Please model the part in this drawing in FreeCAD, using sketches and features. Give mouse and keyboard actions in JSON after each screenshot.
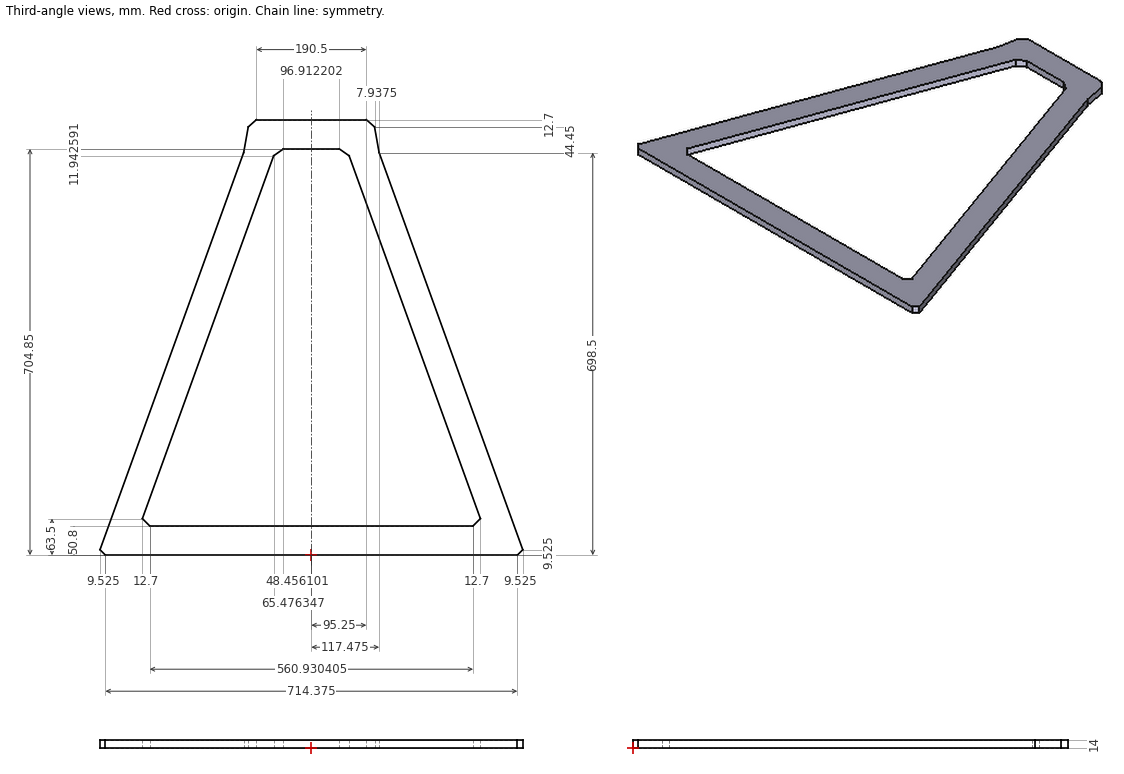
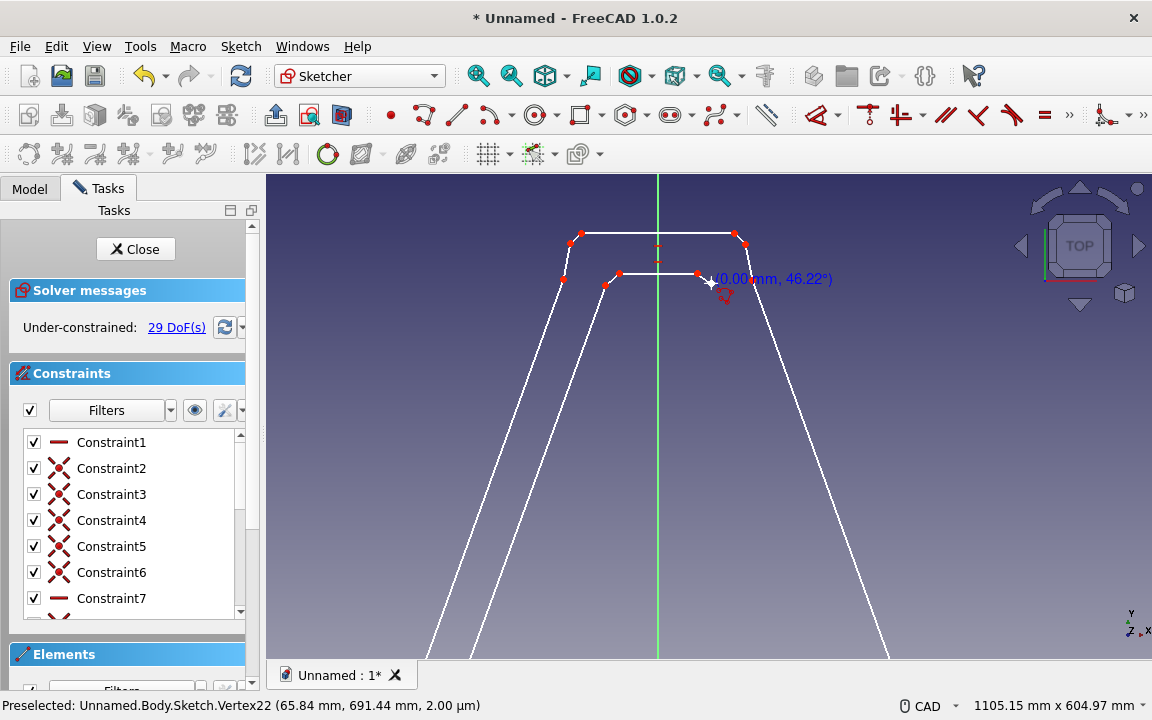
{"action": "scroll", "coordinate": [619, 272], "scroll_direction": "down", "scroll_amount": 3}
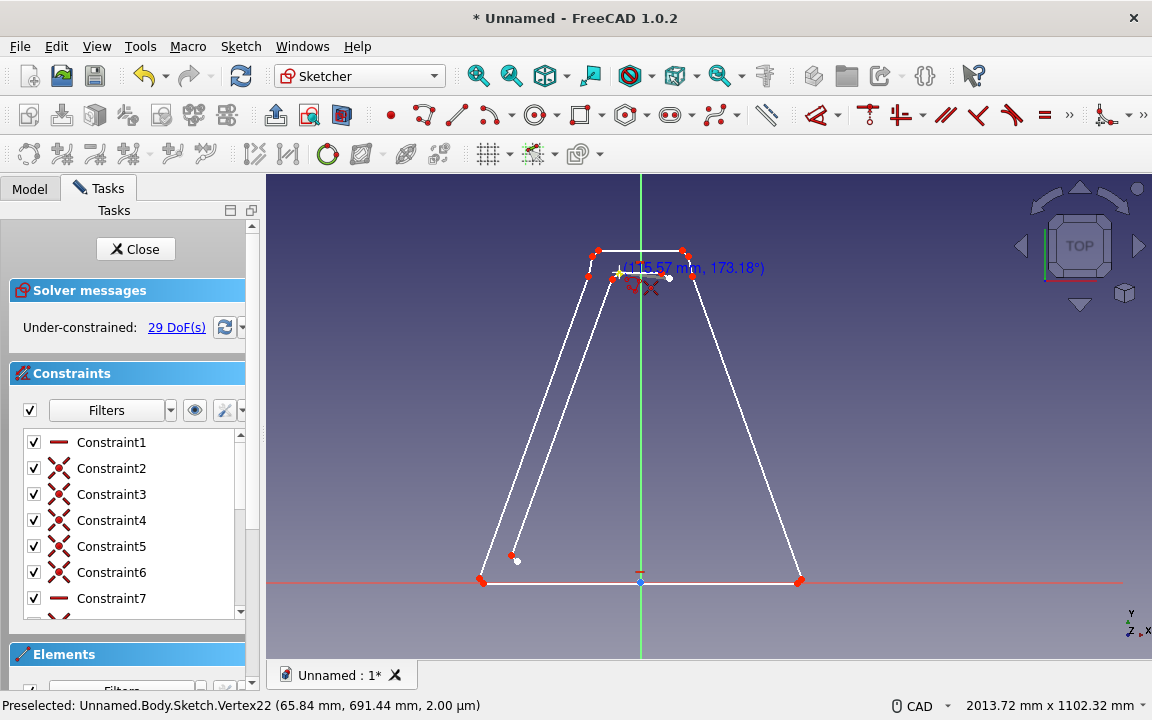
{"action": "left_click", "coordinate": [770, 555]}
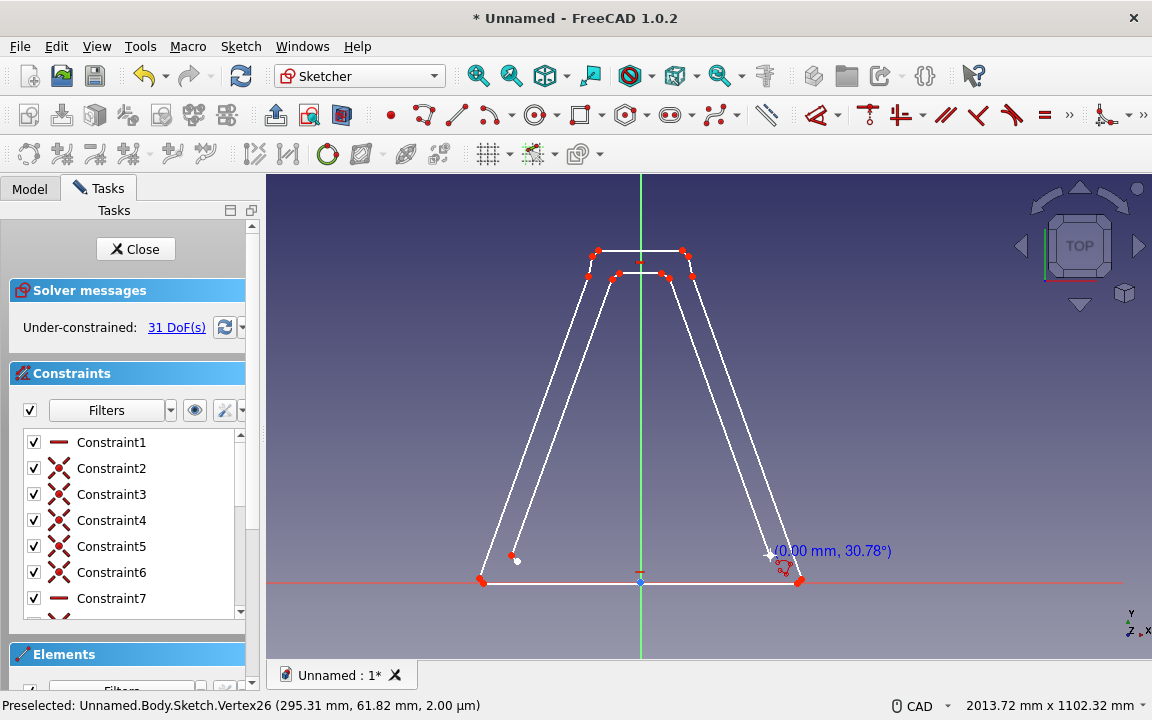
{"action": "scroll", "coordinate": [764, 561], "scroll_direction": "up", "scroll_amount": 4}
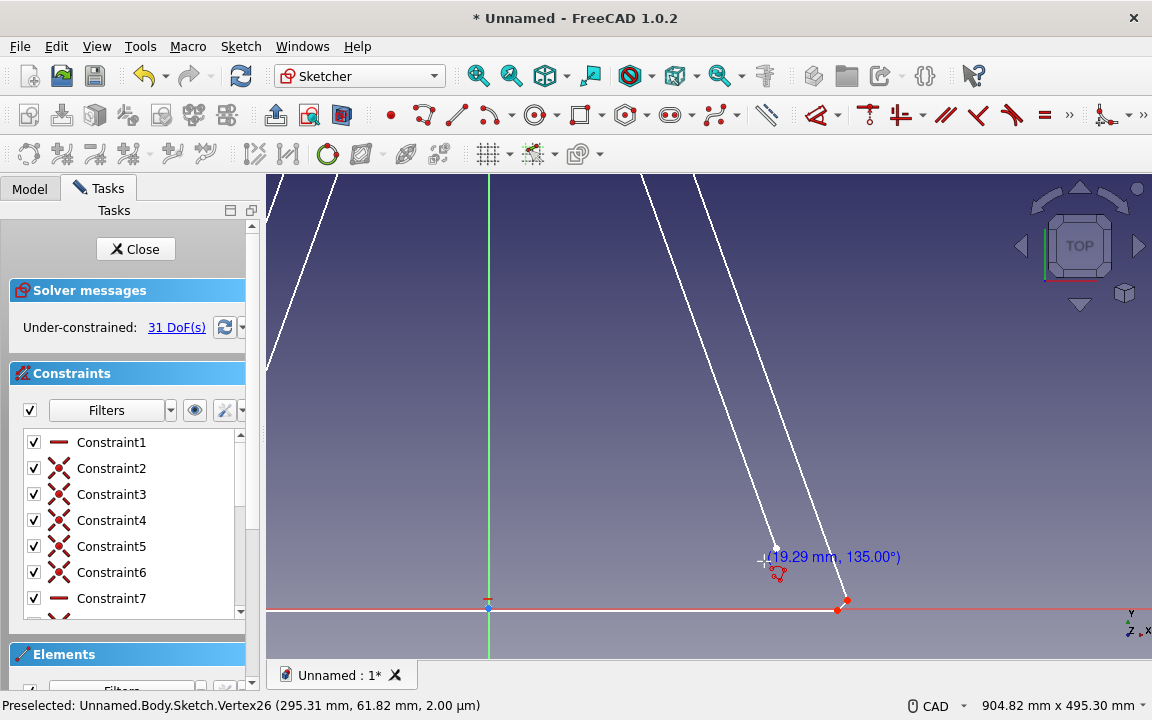
{"action": "left_click", "coordinate": [763, 559]}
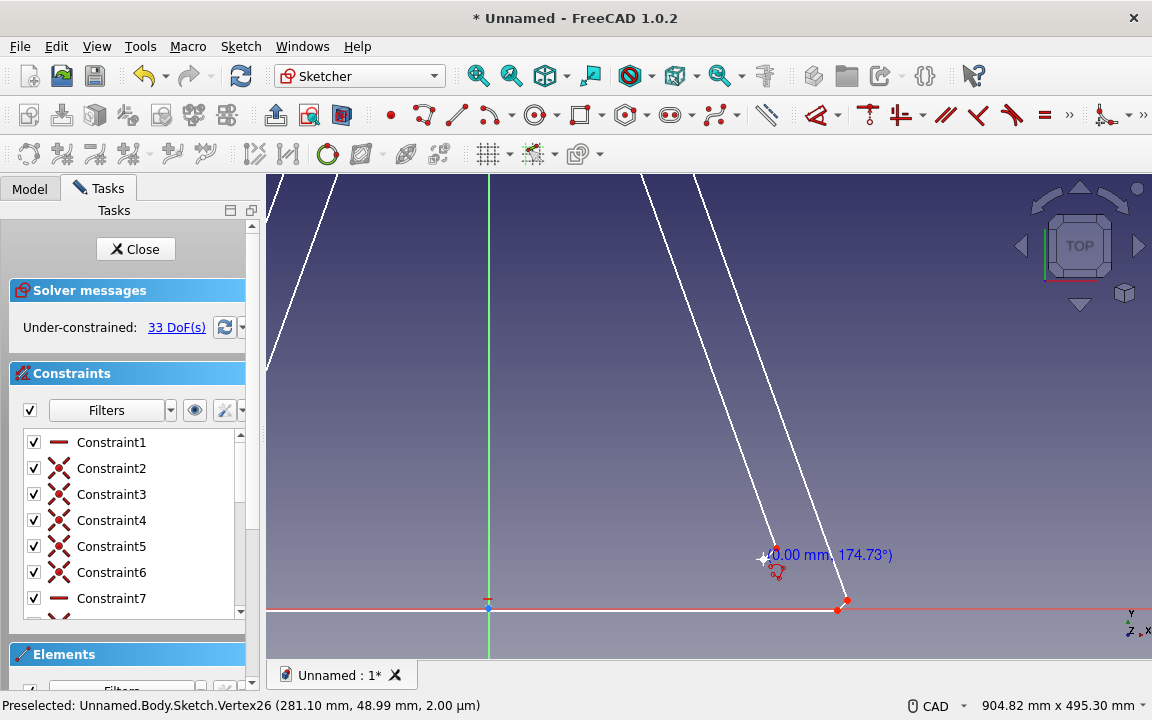
{"action": "scroll", "coordinate": [764, 561], "scroll_direction": "down", "scroll_amount": 4}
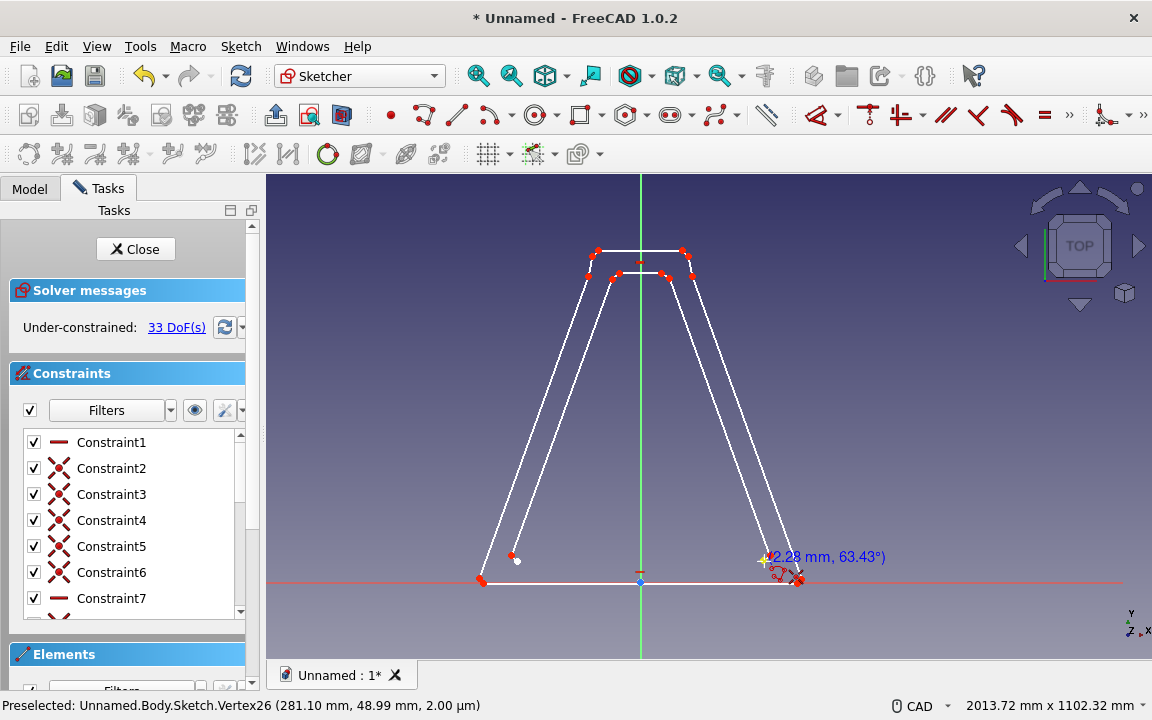
{"action": "scroll", "coordinate": [517, 561], "scroll_direction": "up", "scroll_amount": 7}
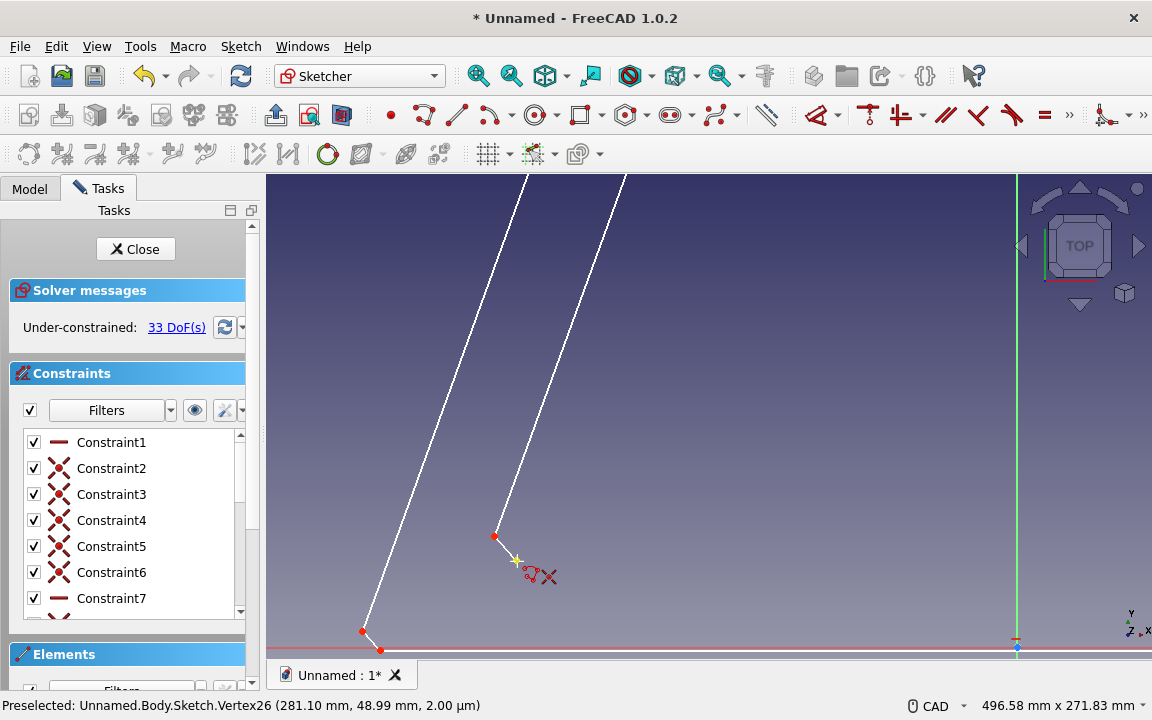
{"action": "left_click", "coordinate": [516, 561]}
{"action": "key", "text": "Escape"}
{"action": "key", "text": "Escape"}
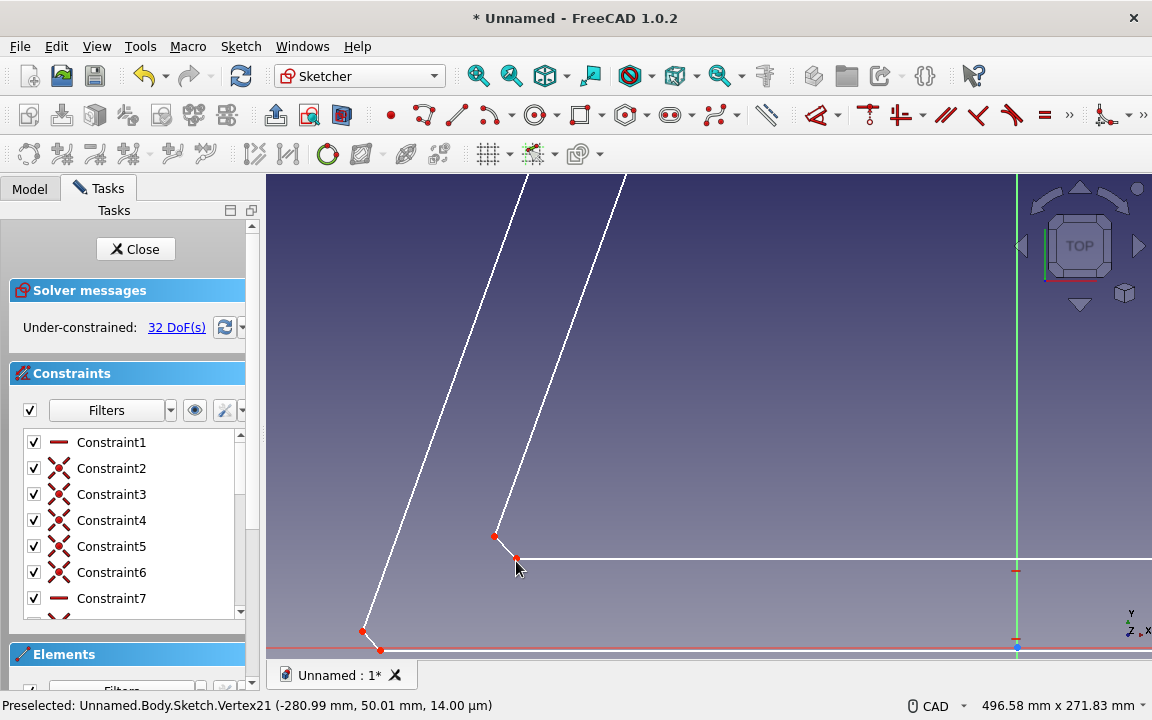
{"action": "scroll", "coordinate": [517, 561], "scroll_direction": "down", "scroll_amount": 7}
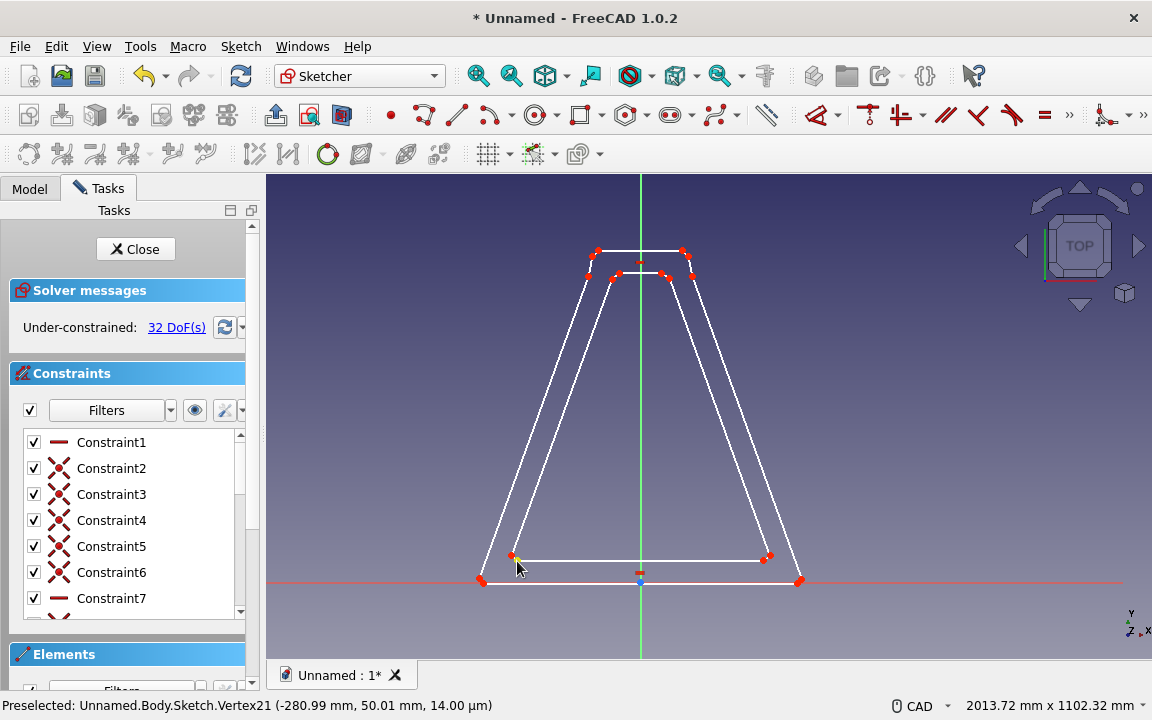
{"action": "scroll", "coordinate": [688, 257], "scroll_direction": "up", "scroll_amount": 2}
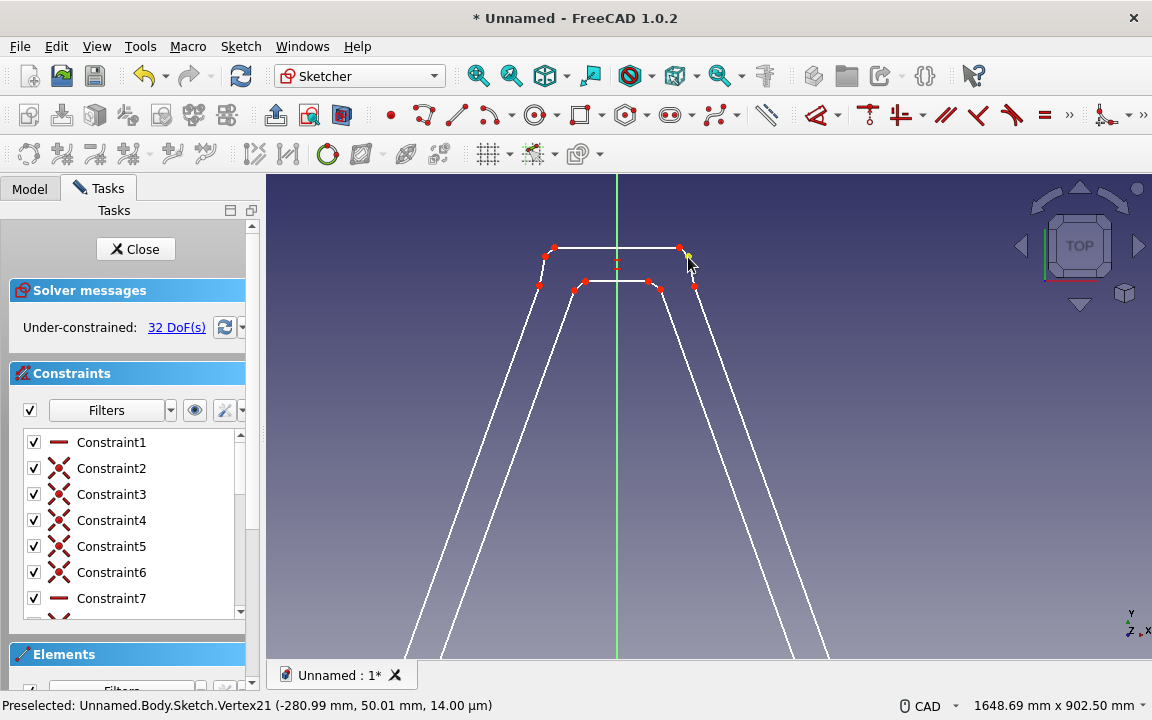
{"action": "left_click", "coordinate": [688, 257]}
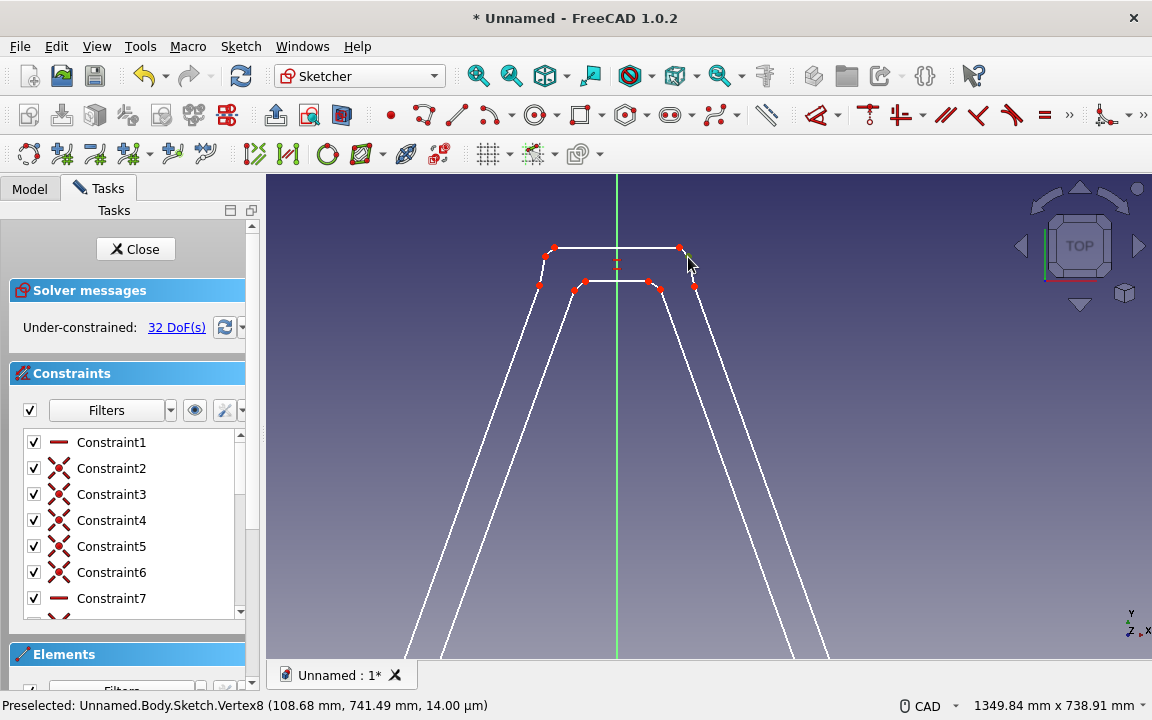
{"action": "left_click", "coordinate": [545, 256]}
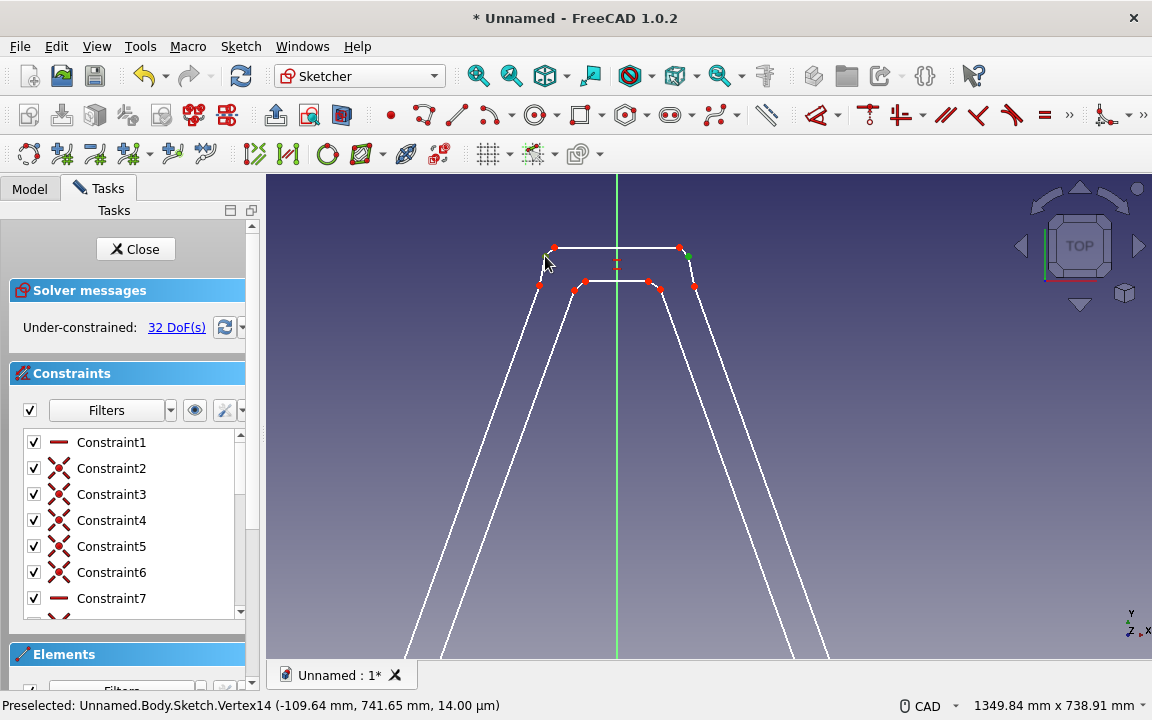
{"action": "left_click", "coordinate": [617, 600]}